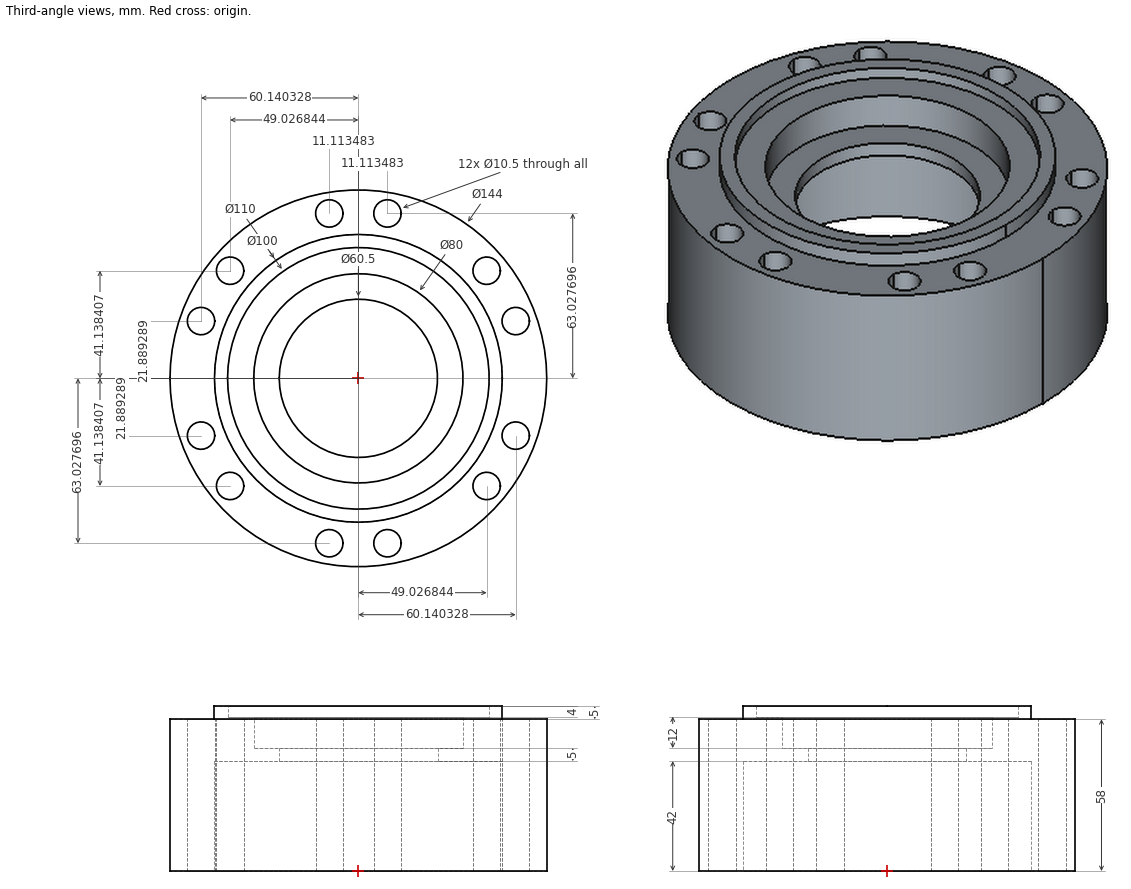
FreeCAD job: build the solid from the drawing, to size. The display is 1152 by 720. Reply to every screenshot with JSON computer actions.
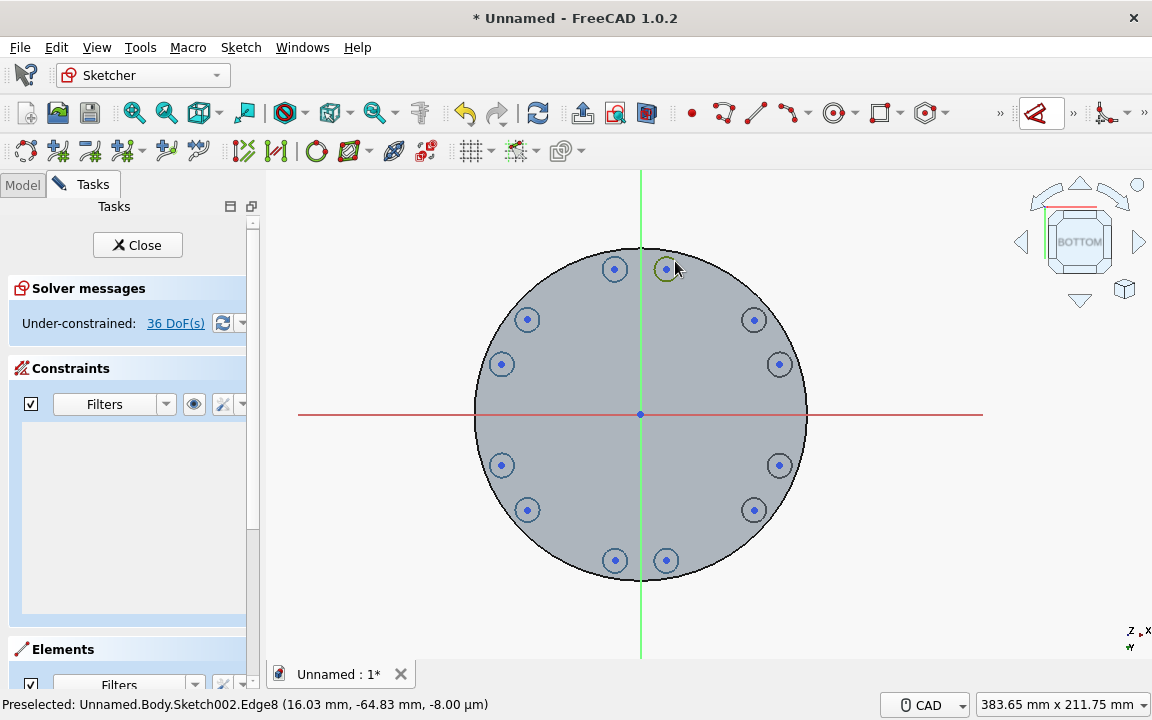
{"action": "left_click", "coordinate": [763, 312]}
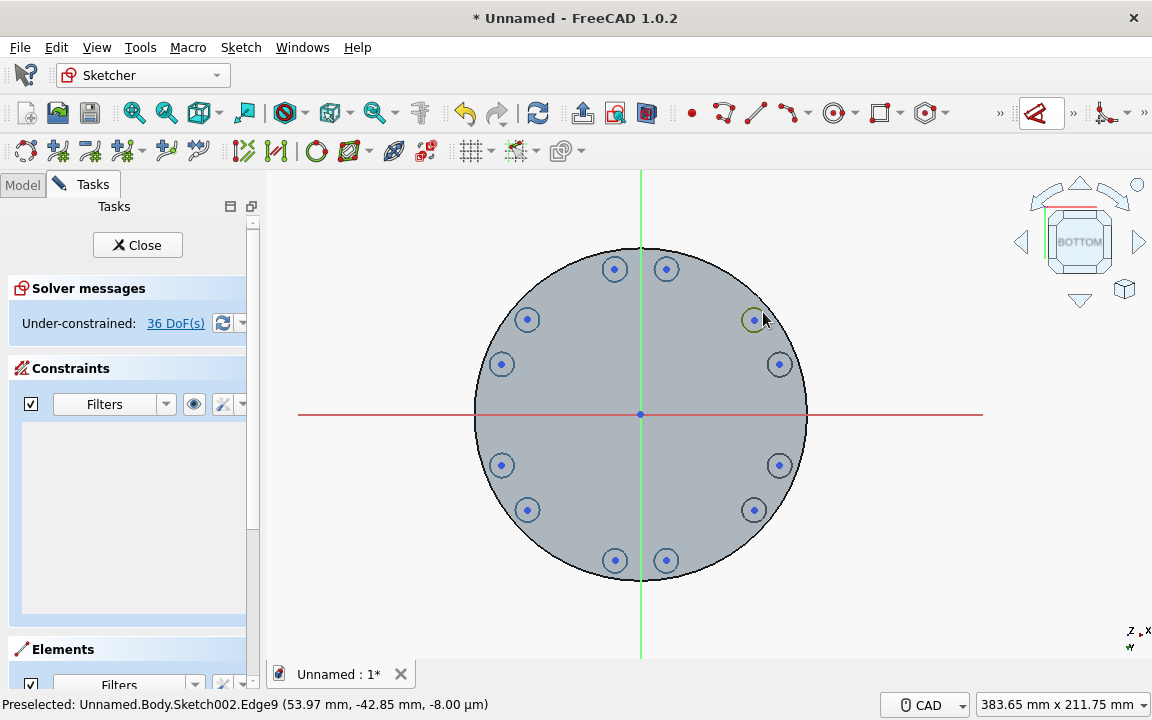
{"action": "left_click", "coordinate": [788, 356]}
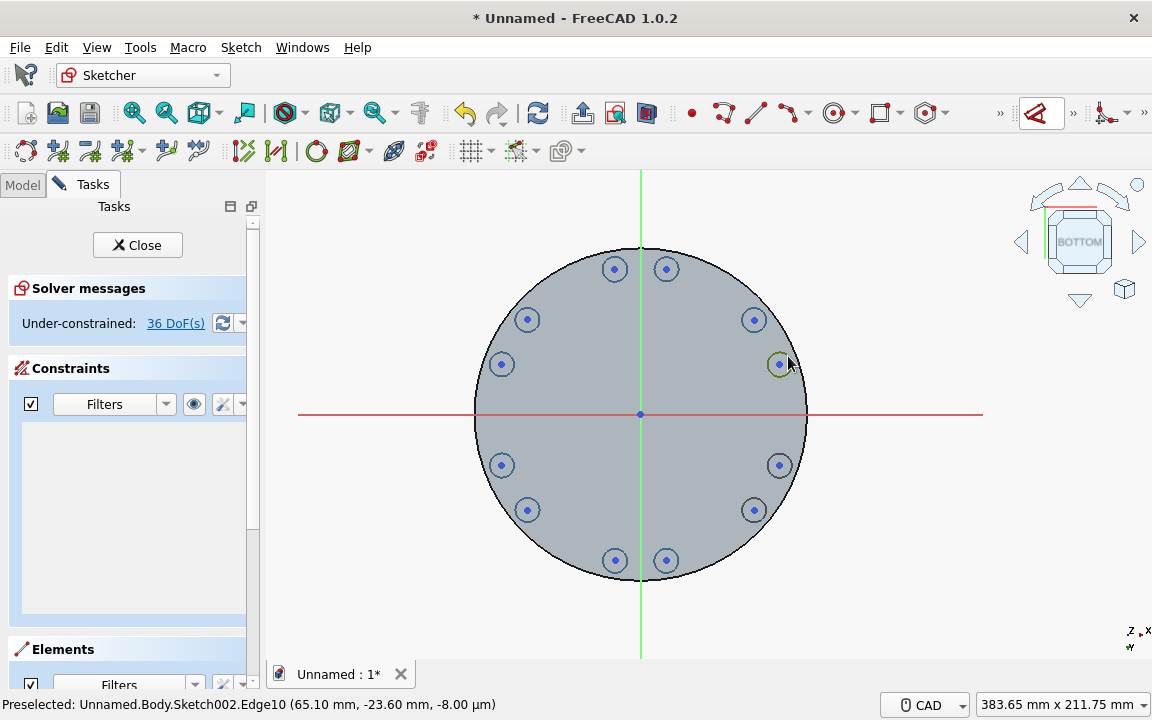
{"action": "left_click", "coordinate": [788, 457]}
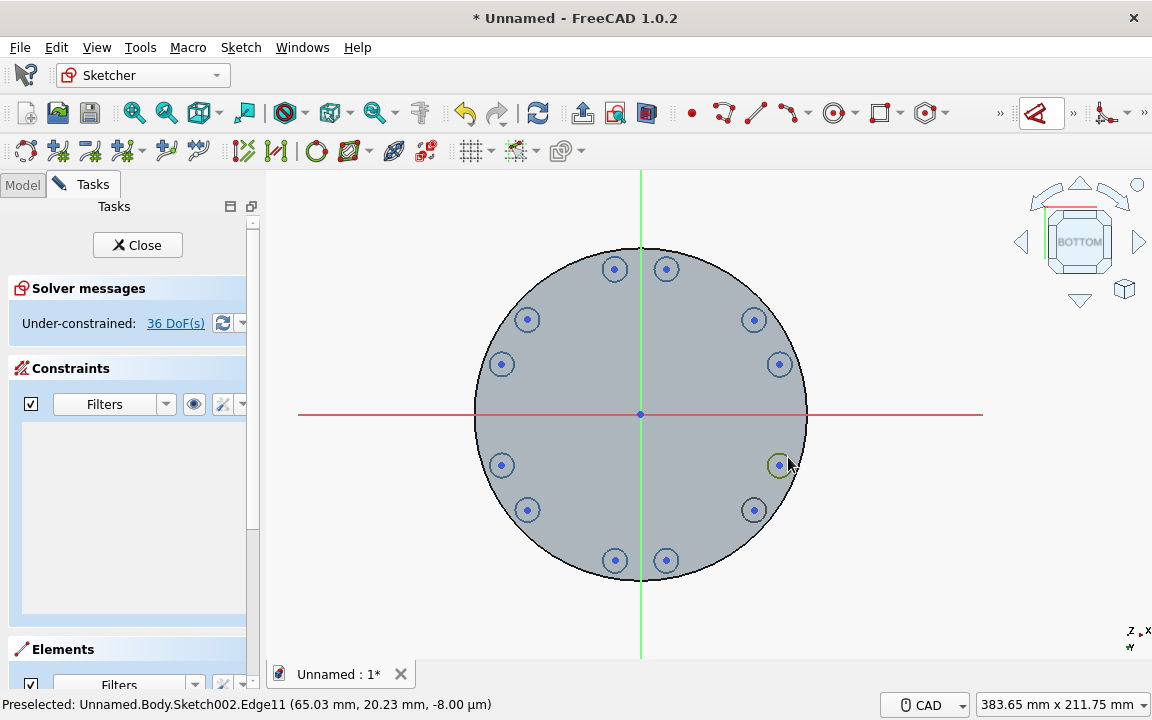
{"action": "left_click", "coordinate": [763, 502]}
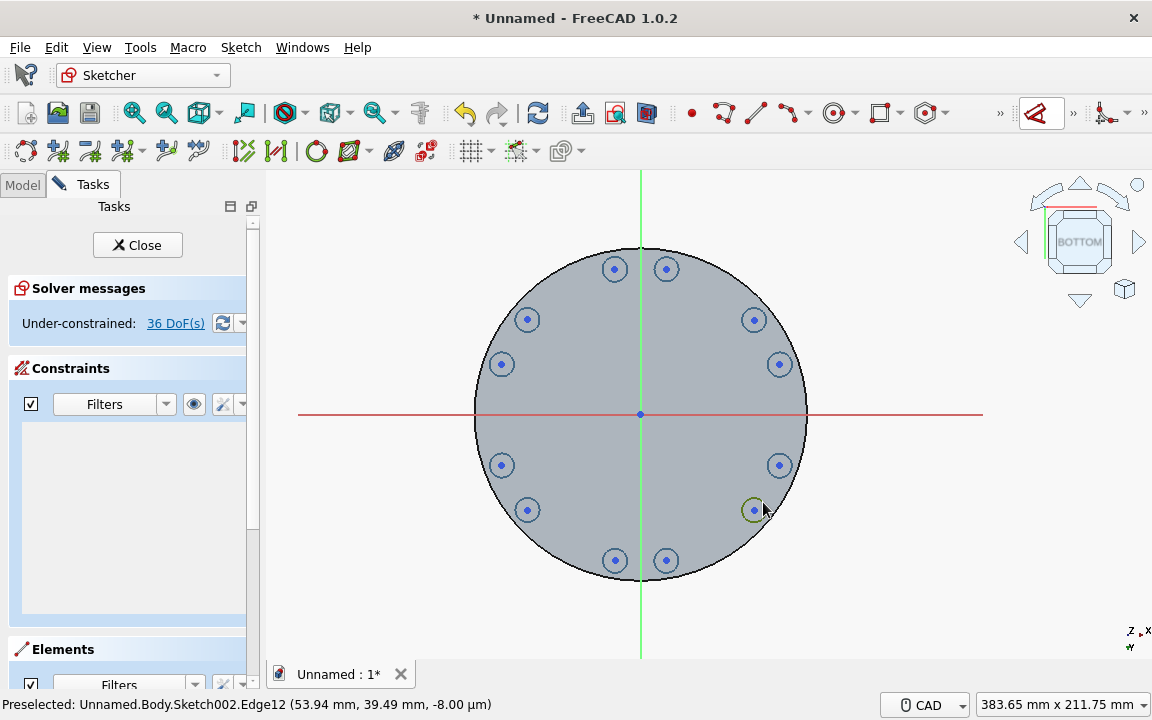
{"action": "key", "text": "e"}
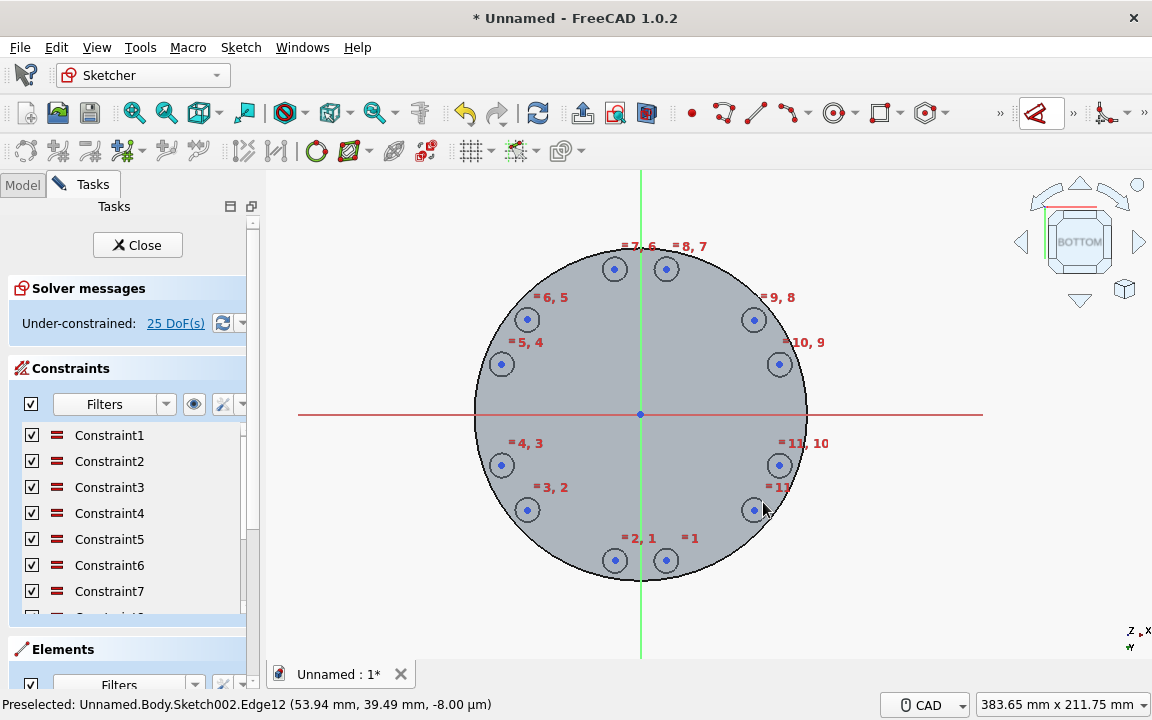
{"action": "left_click", "coordinate": [666, 561]}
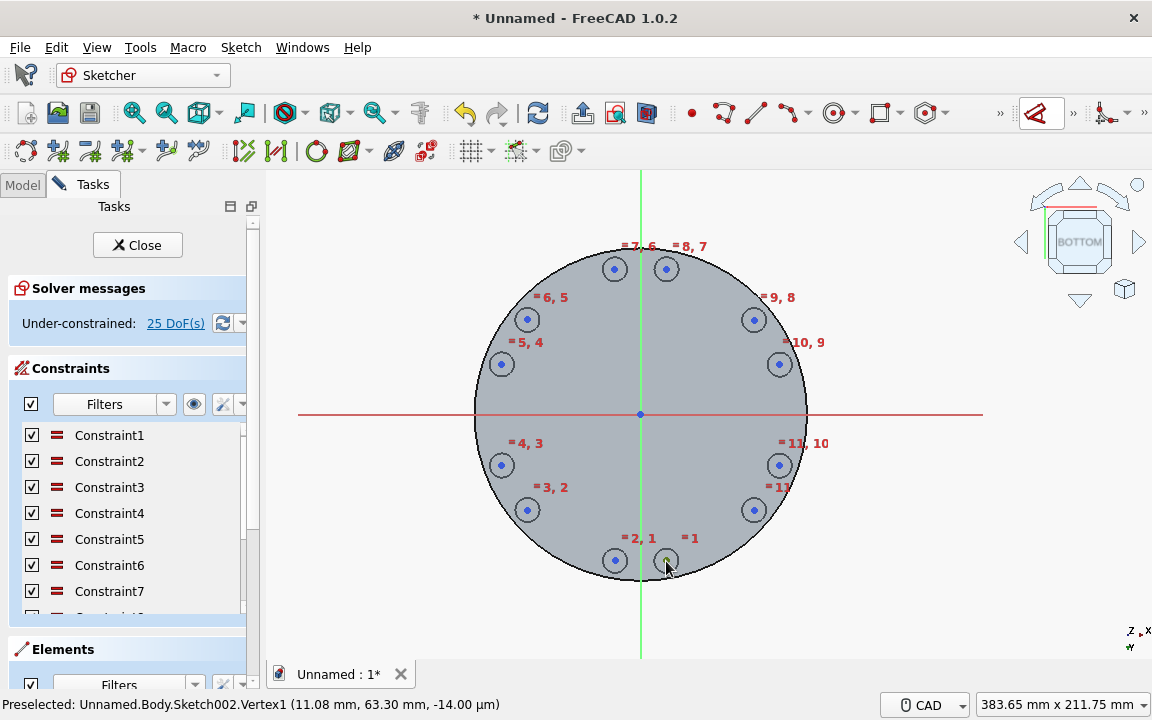
{"action": "left_click", "coordinate": [615, 561]}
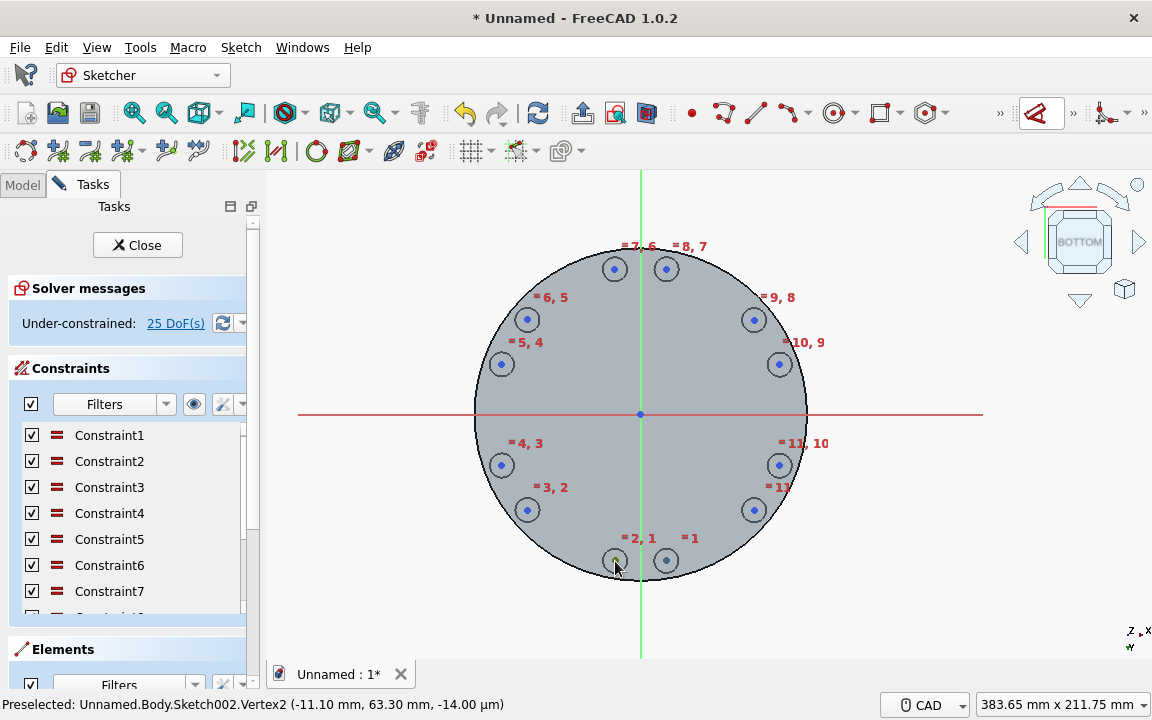
{"action": "key", "text": "h"}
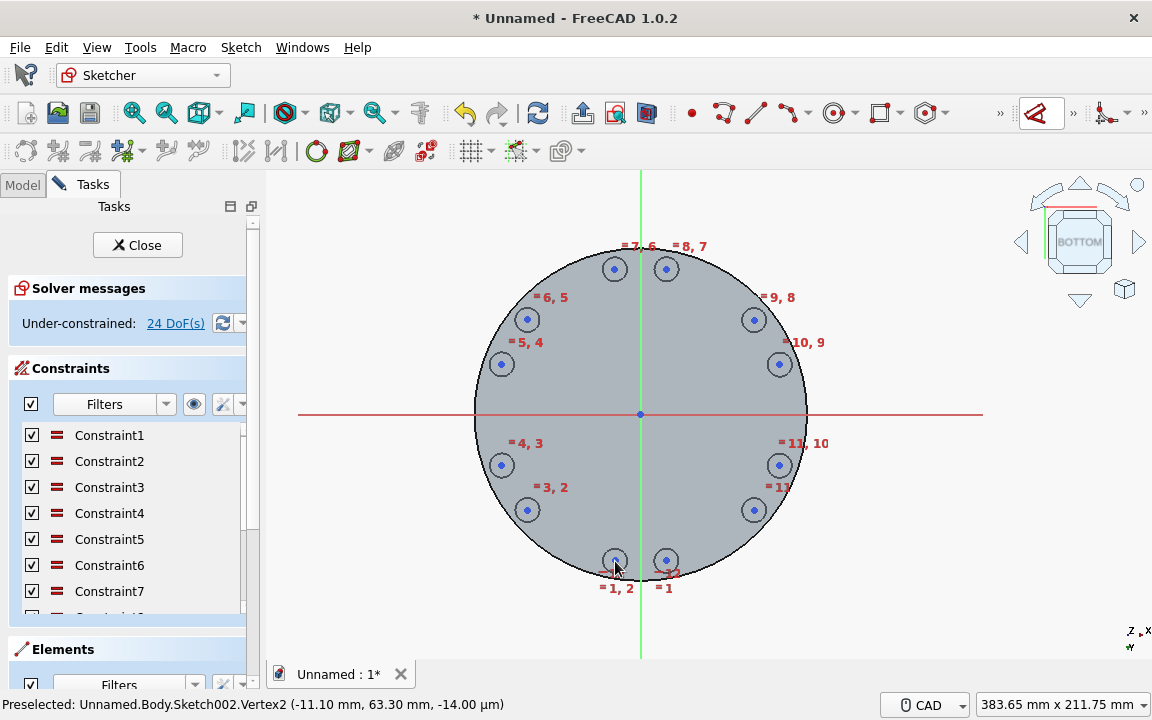
{"action": "left_click", "coordinate": [502, 466]}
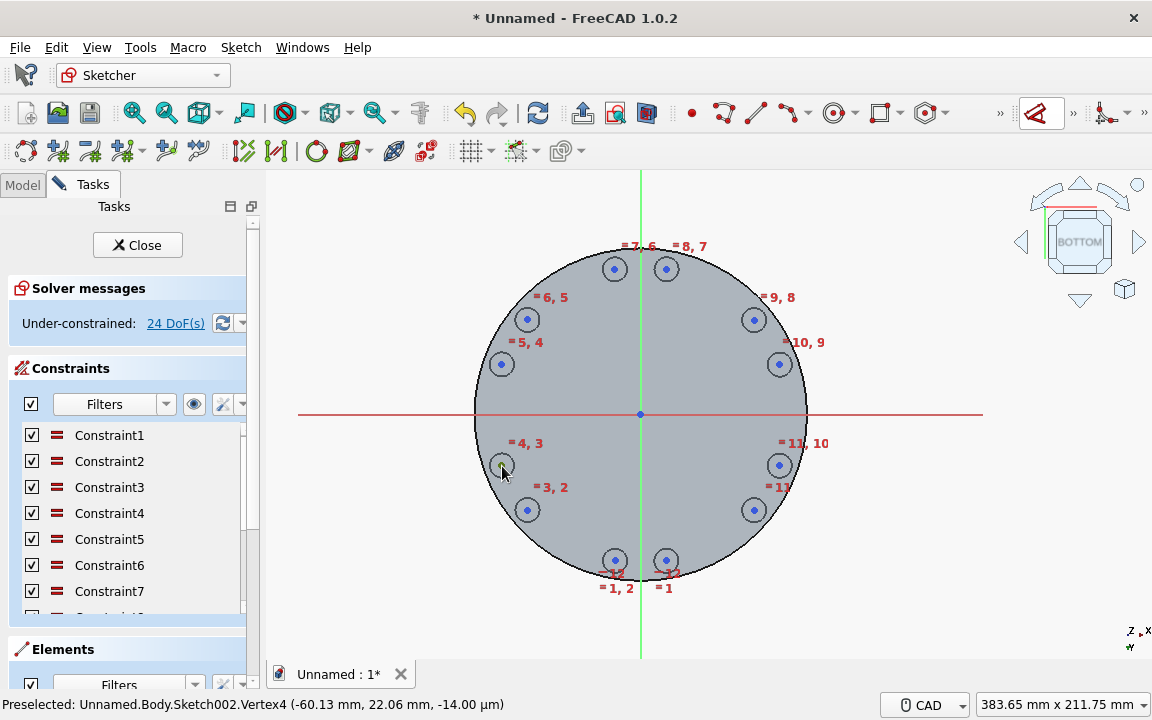
{"action": "left_click", "coordinate": [502, 364]}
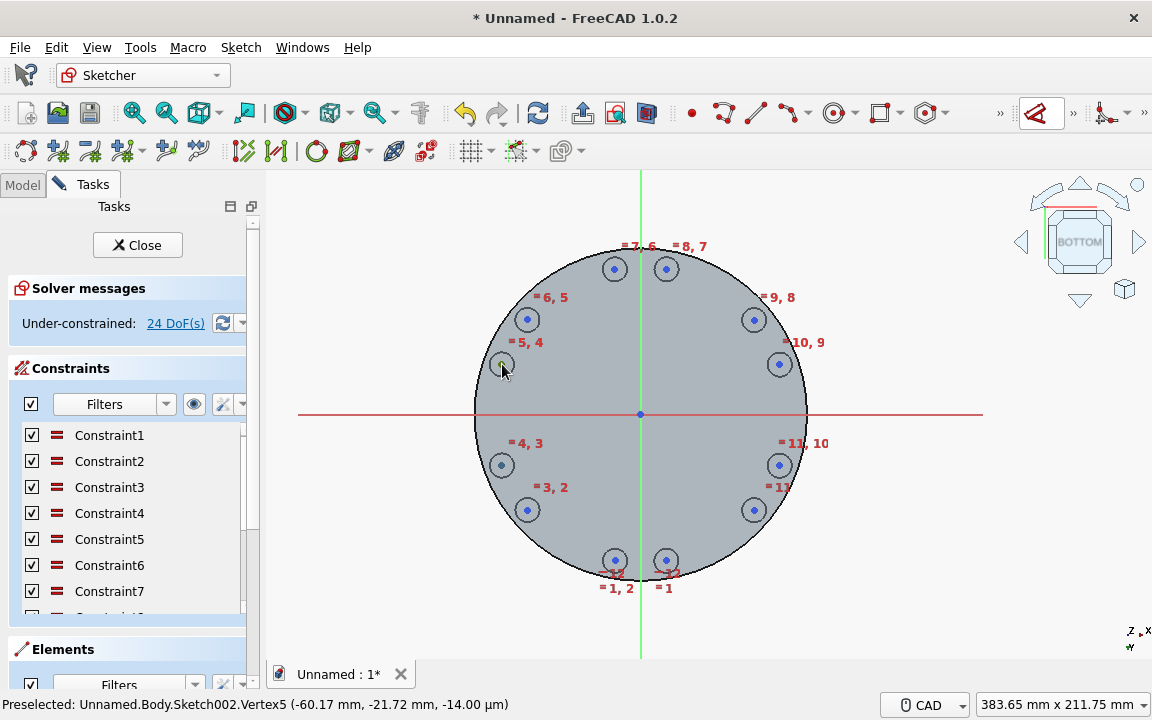
{"action": "key", "text": "v"}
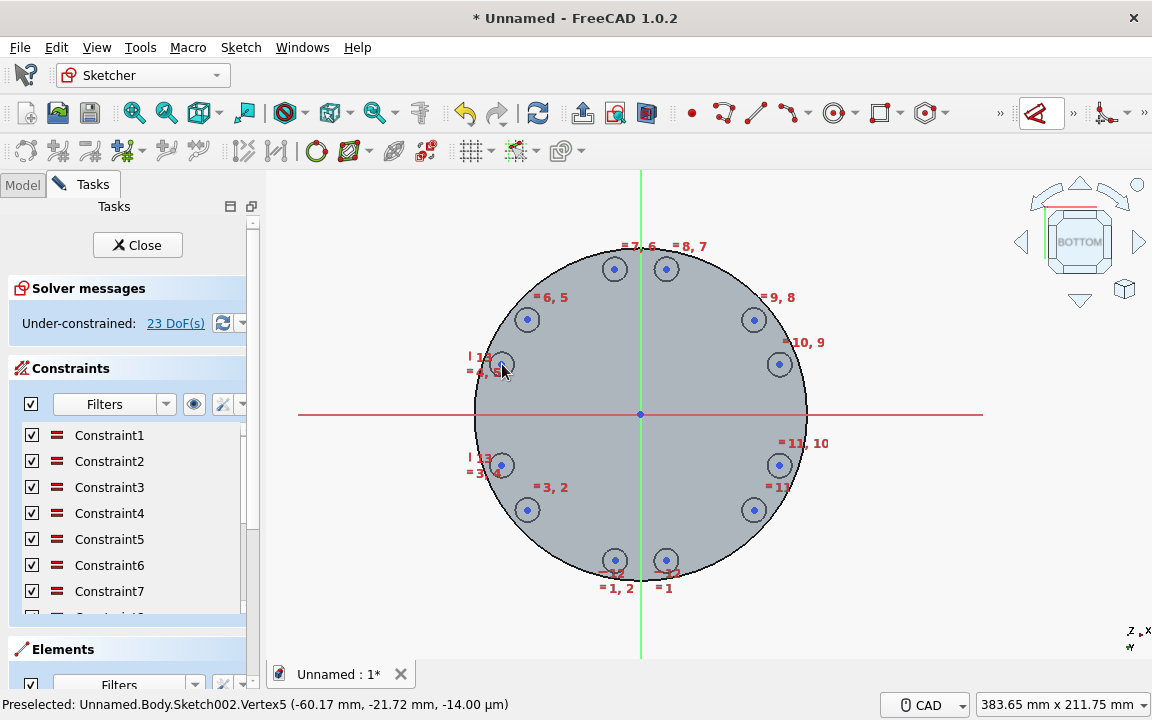
{"action": "left_click", "coordinate": [528, 510]}